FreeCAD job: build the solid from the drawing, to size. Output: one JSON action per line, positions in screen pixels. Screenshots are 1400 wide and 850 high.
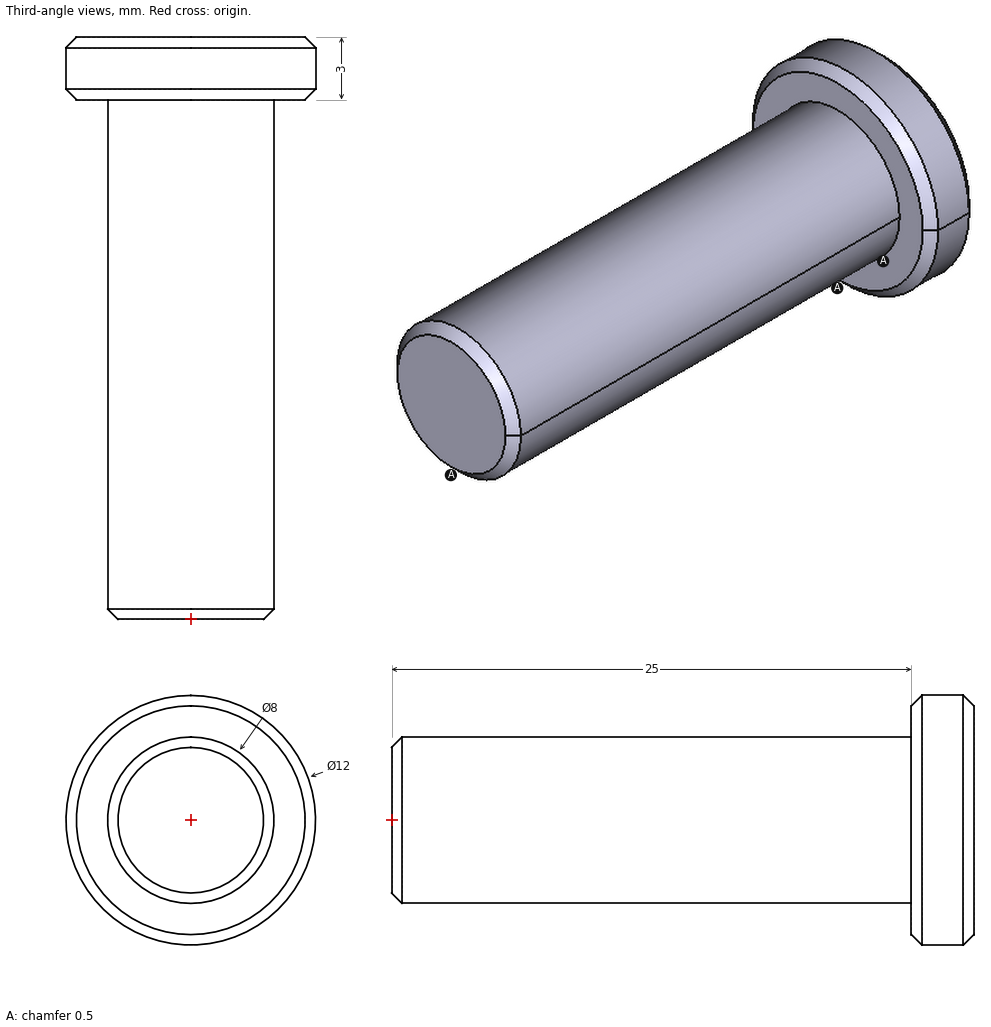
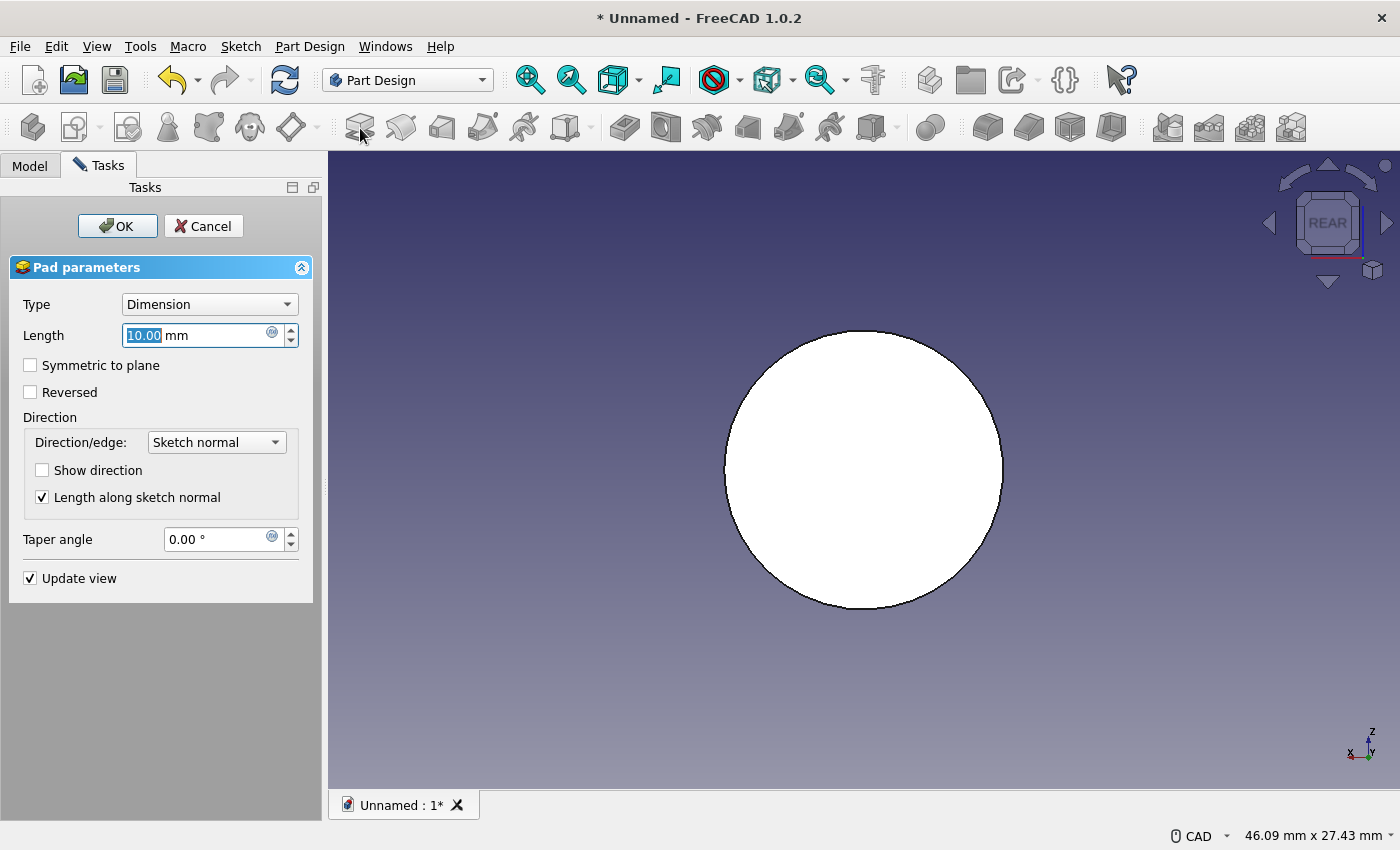
{"action": "type", "text": "3"}
{"action": "key", "text": "Tab"}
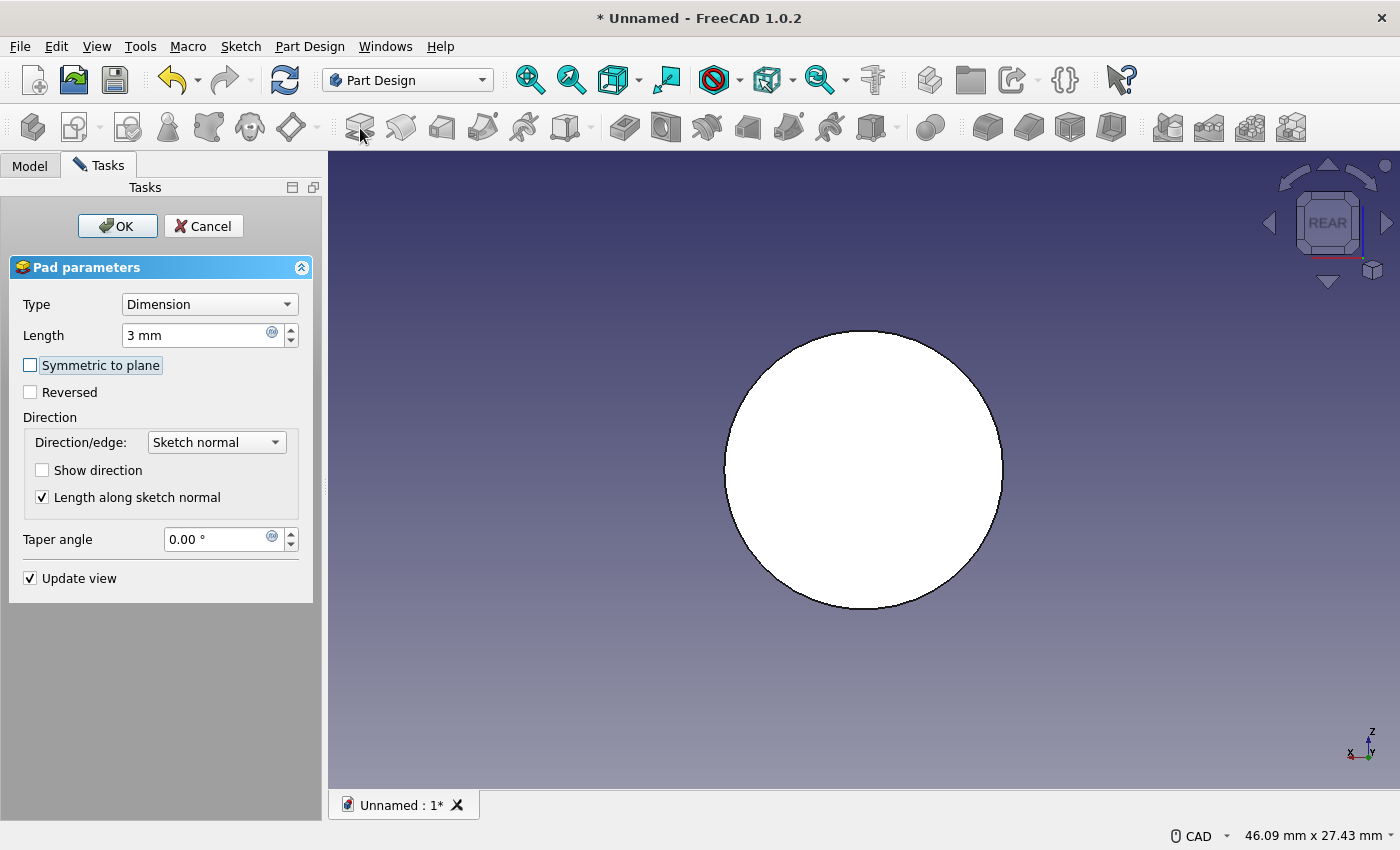
{"action": "left_click", "coordinate": [118, 226]}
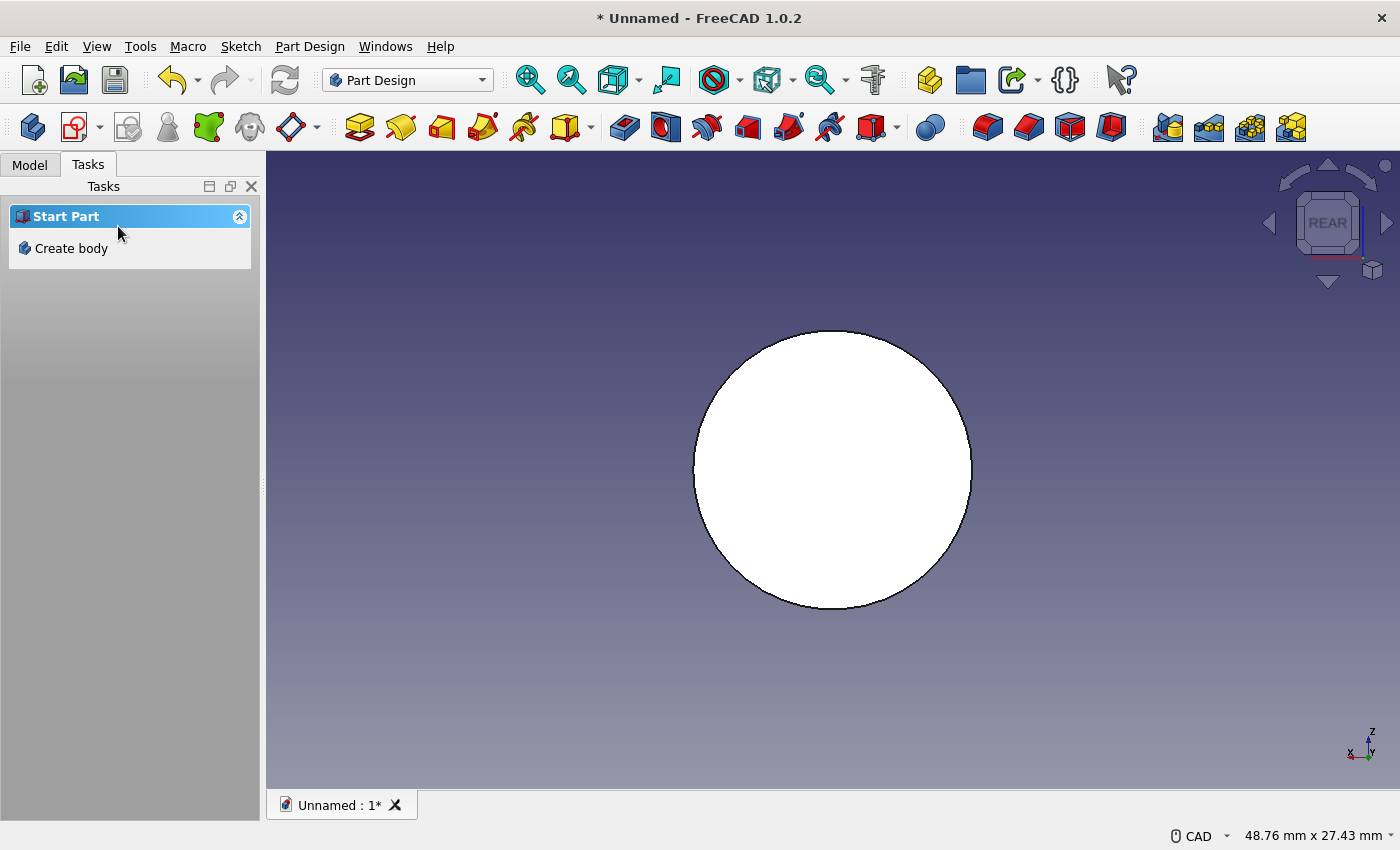
{"action": "key", "text": "v f"}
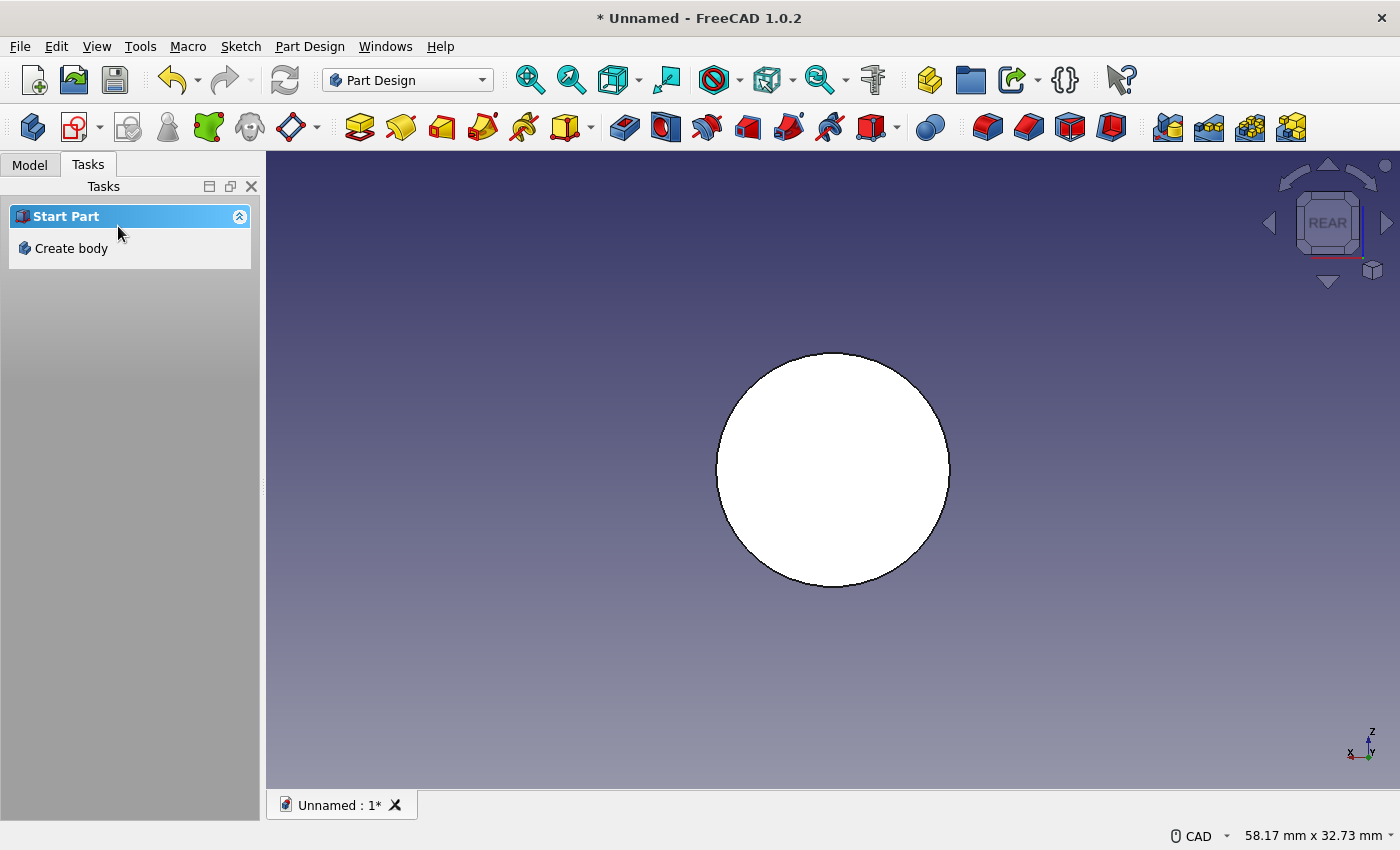
{"action": "left_click", "coordinate": [950, 469]}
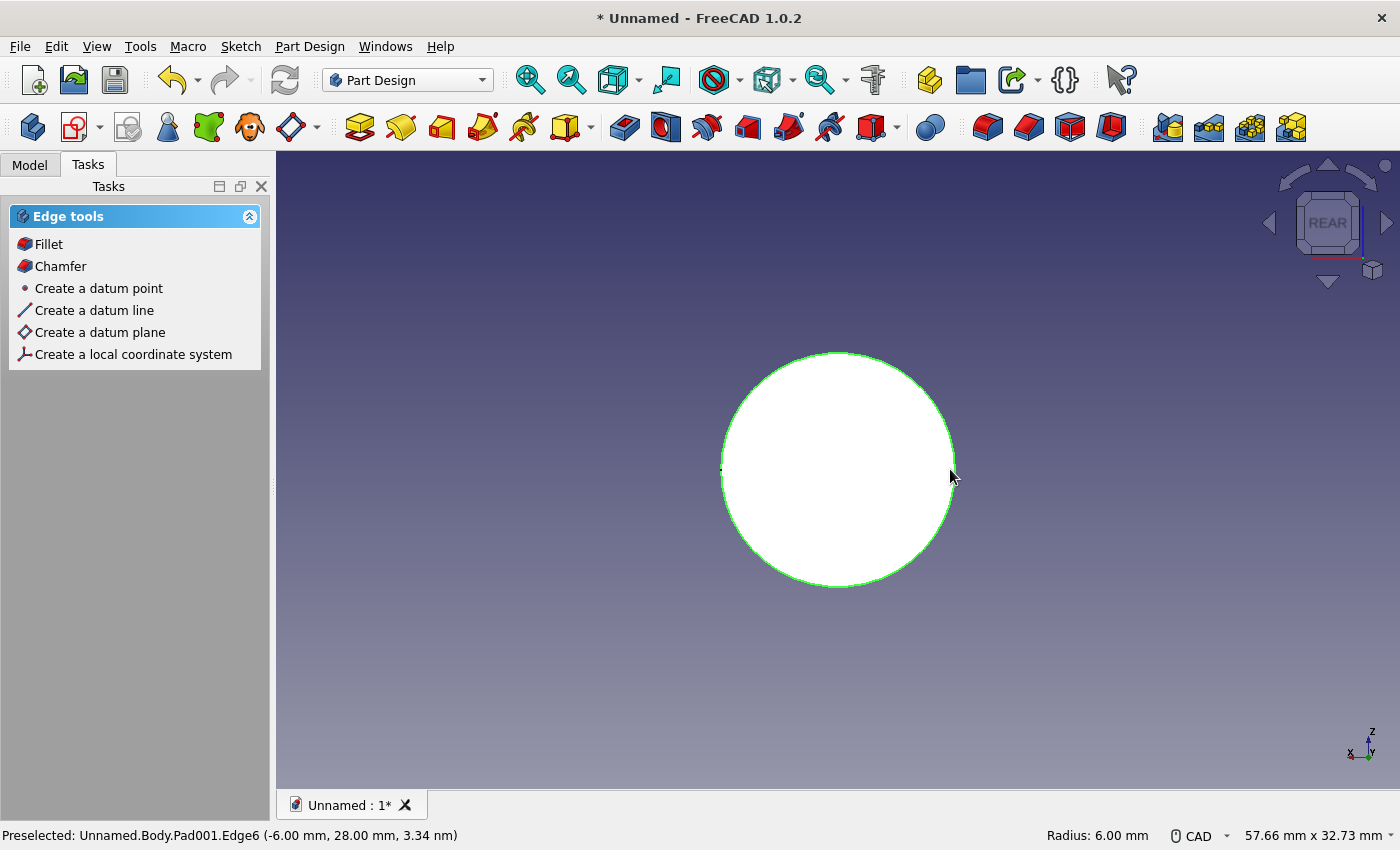
{"action": "key", "text": "0"}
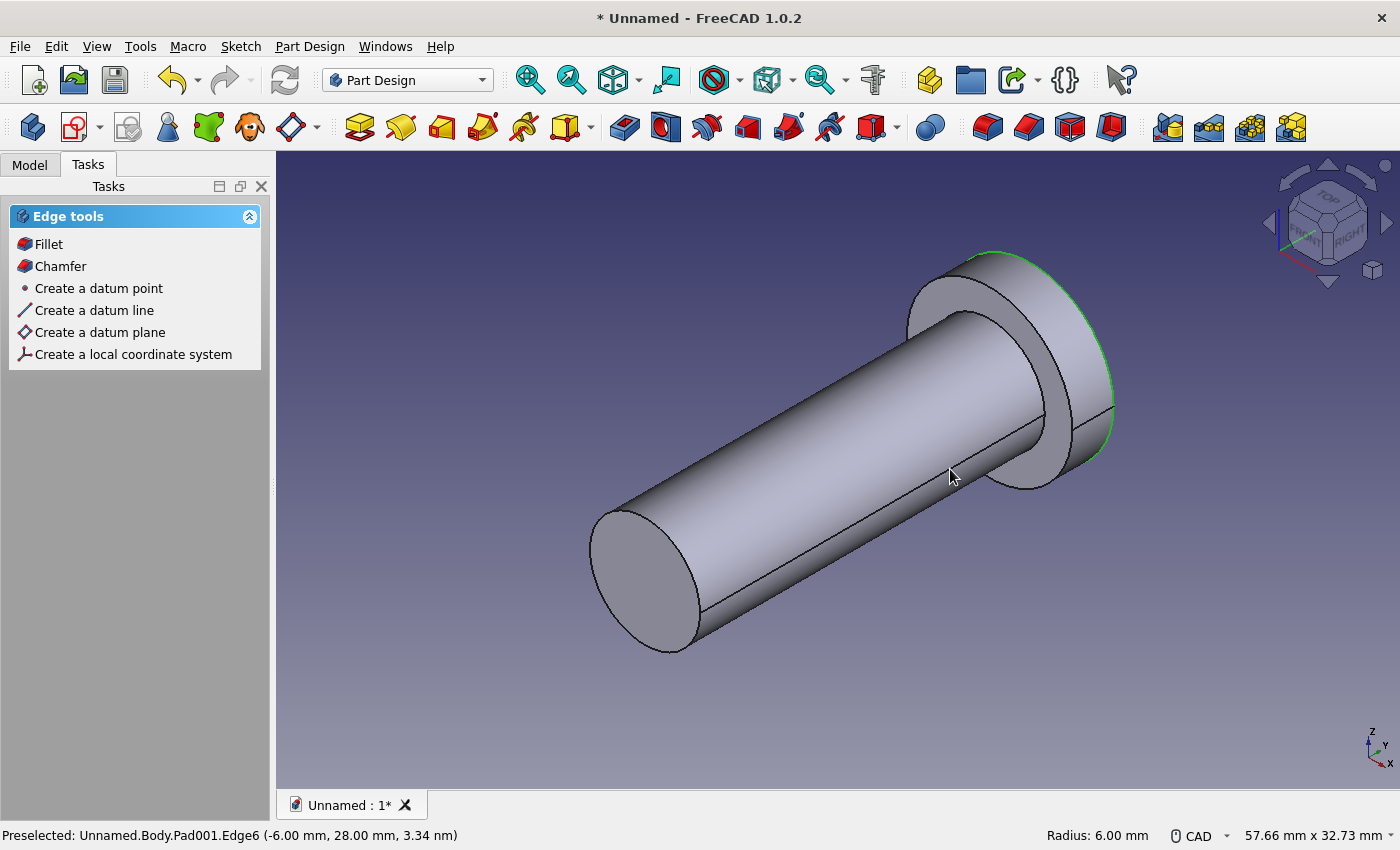
{"action": "left_click", "coordinate": [628, 510], "text": "ctrl"}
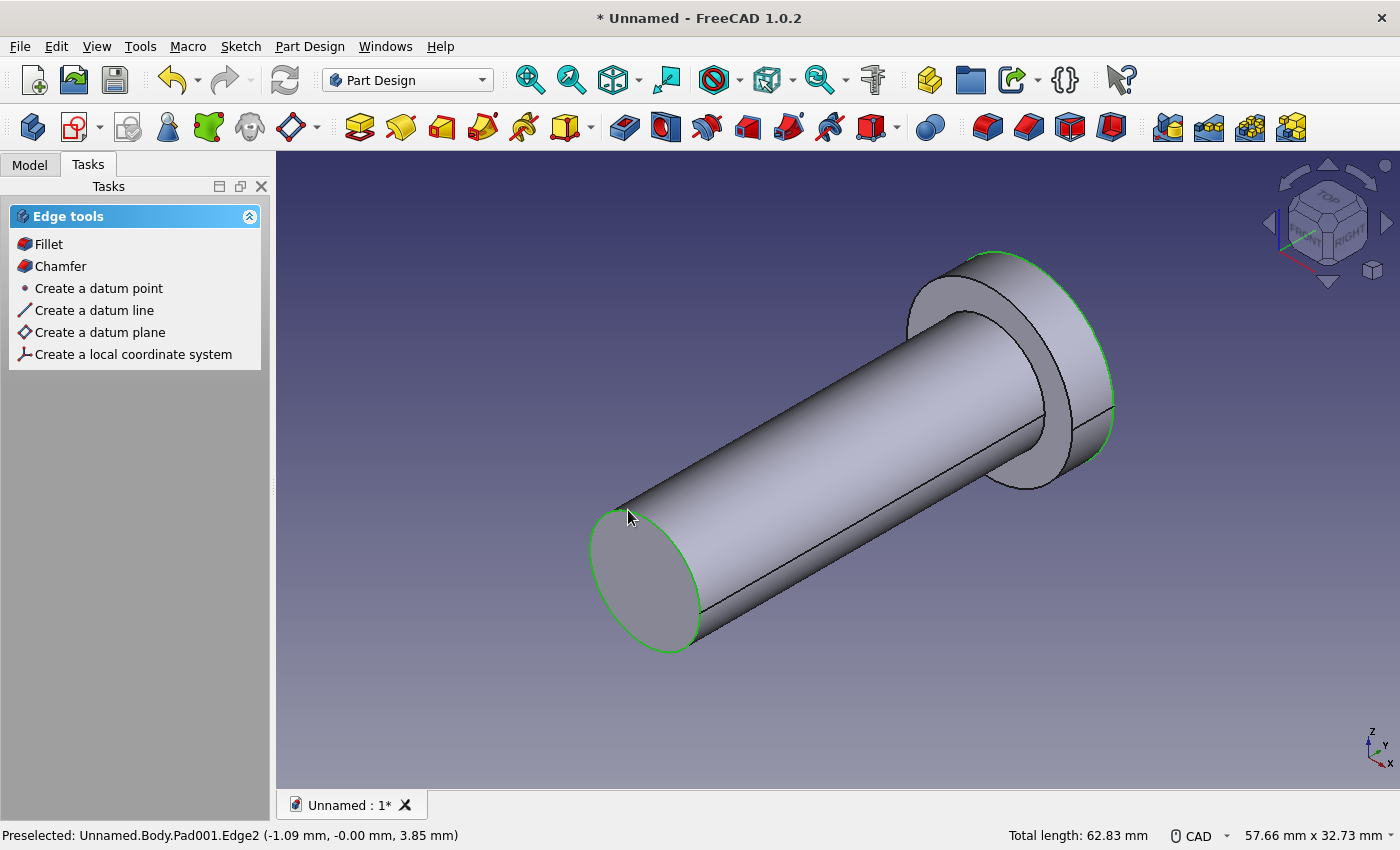
{"action": "left_click", "coordinate": [964, 276], "text": "ctrl"}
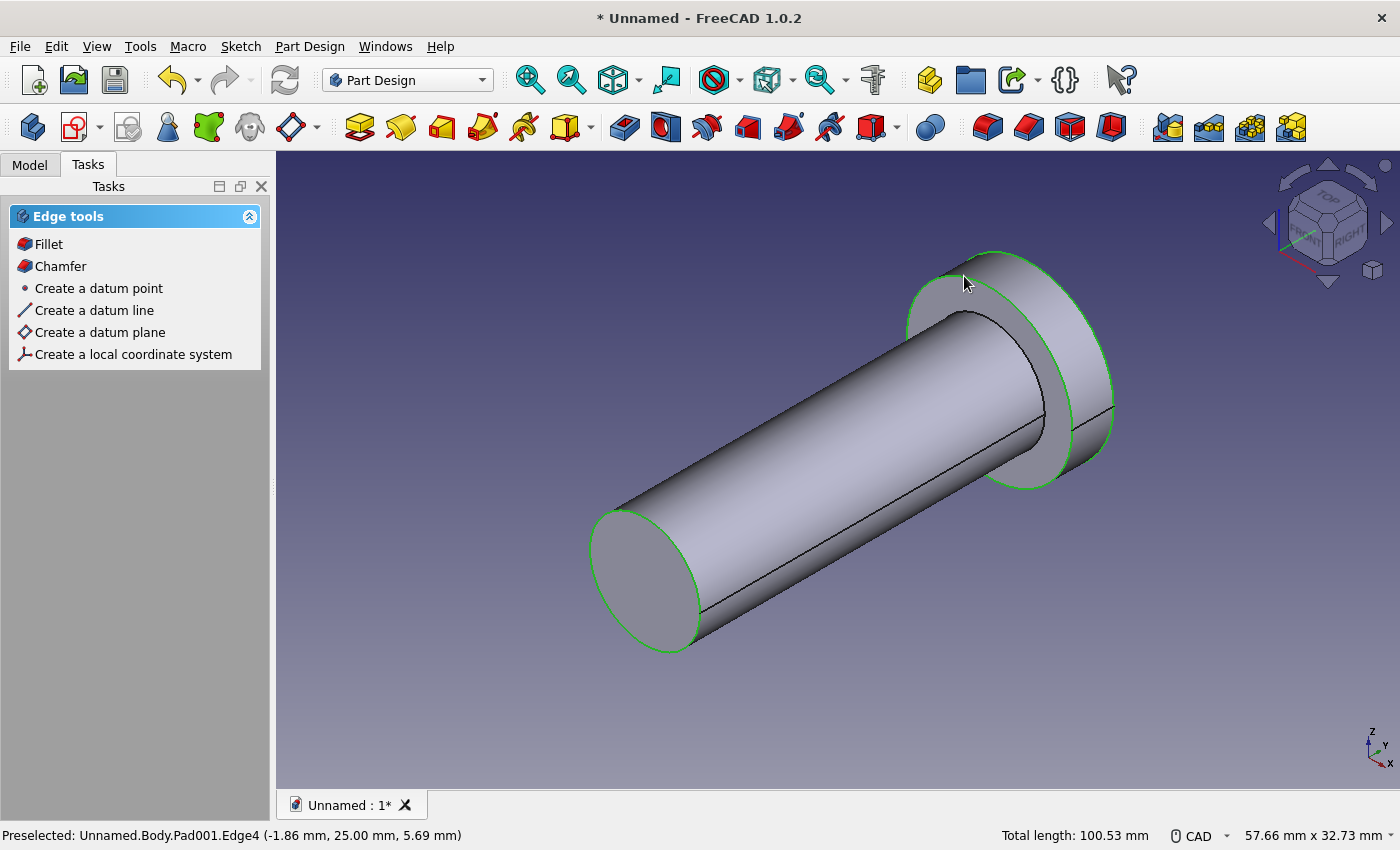
{"action": "left_click", "coordinate": [1029, 128]}